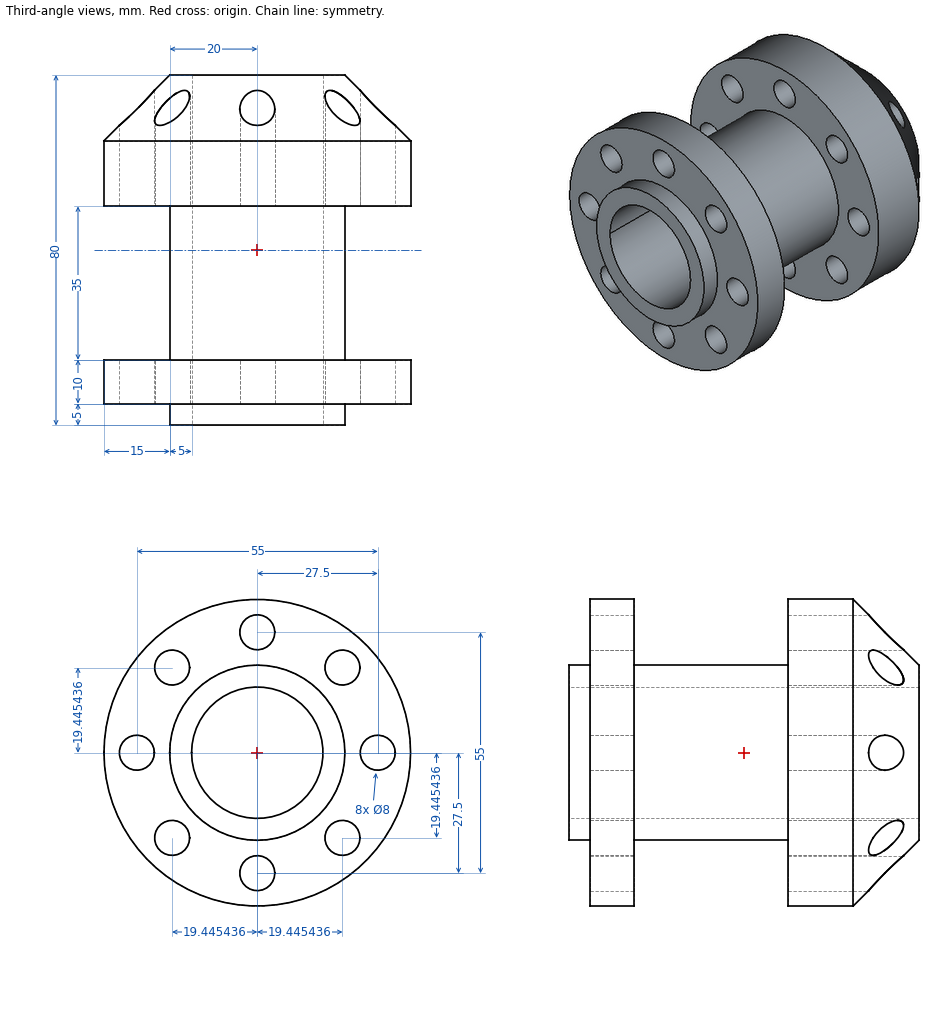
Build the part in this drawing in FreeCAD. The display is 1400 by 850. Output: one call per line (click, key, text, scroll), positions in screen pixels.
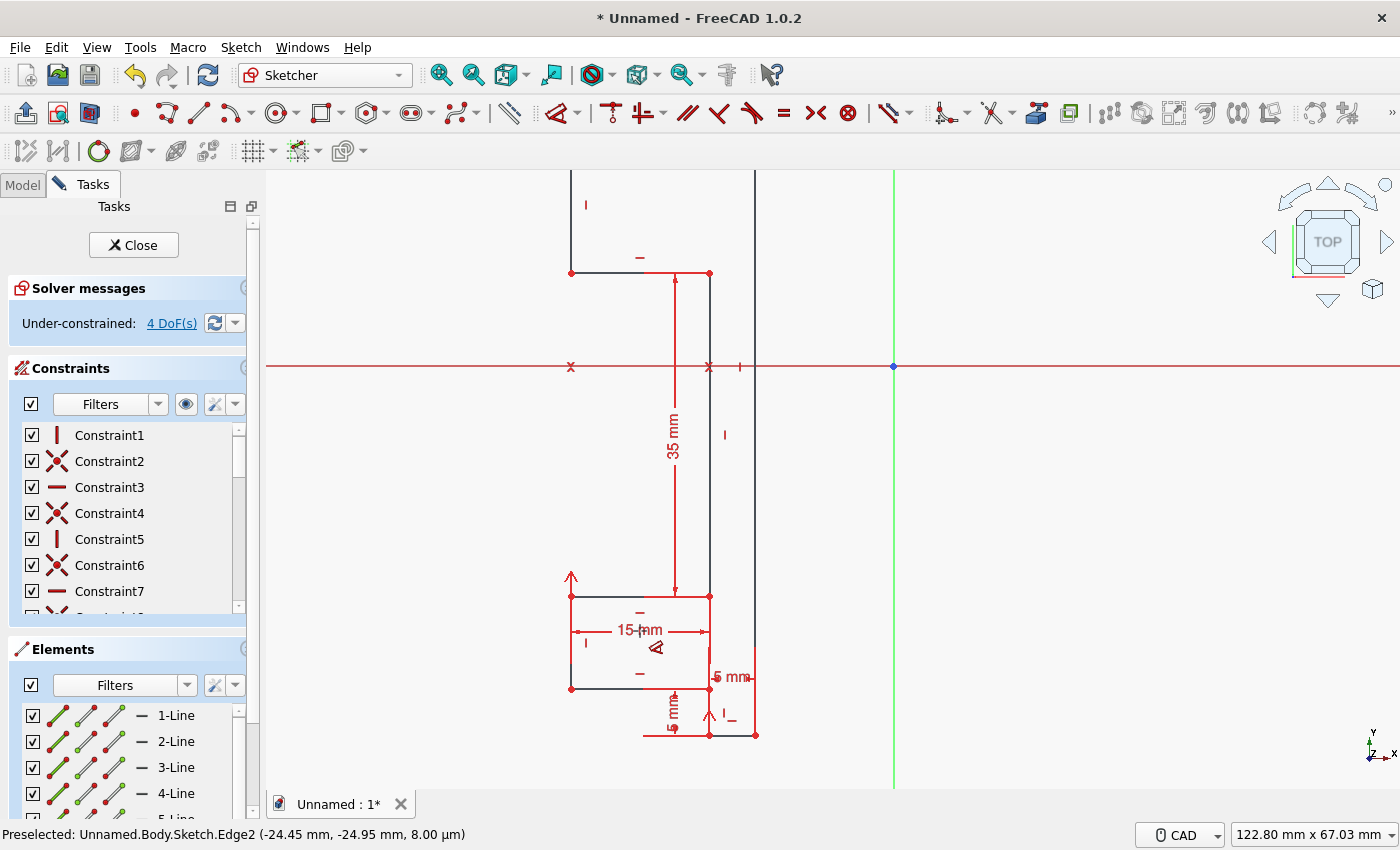
click(571, 624)
click(537, 643)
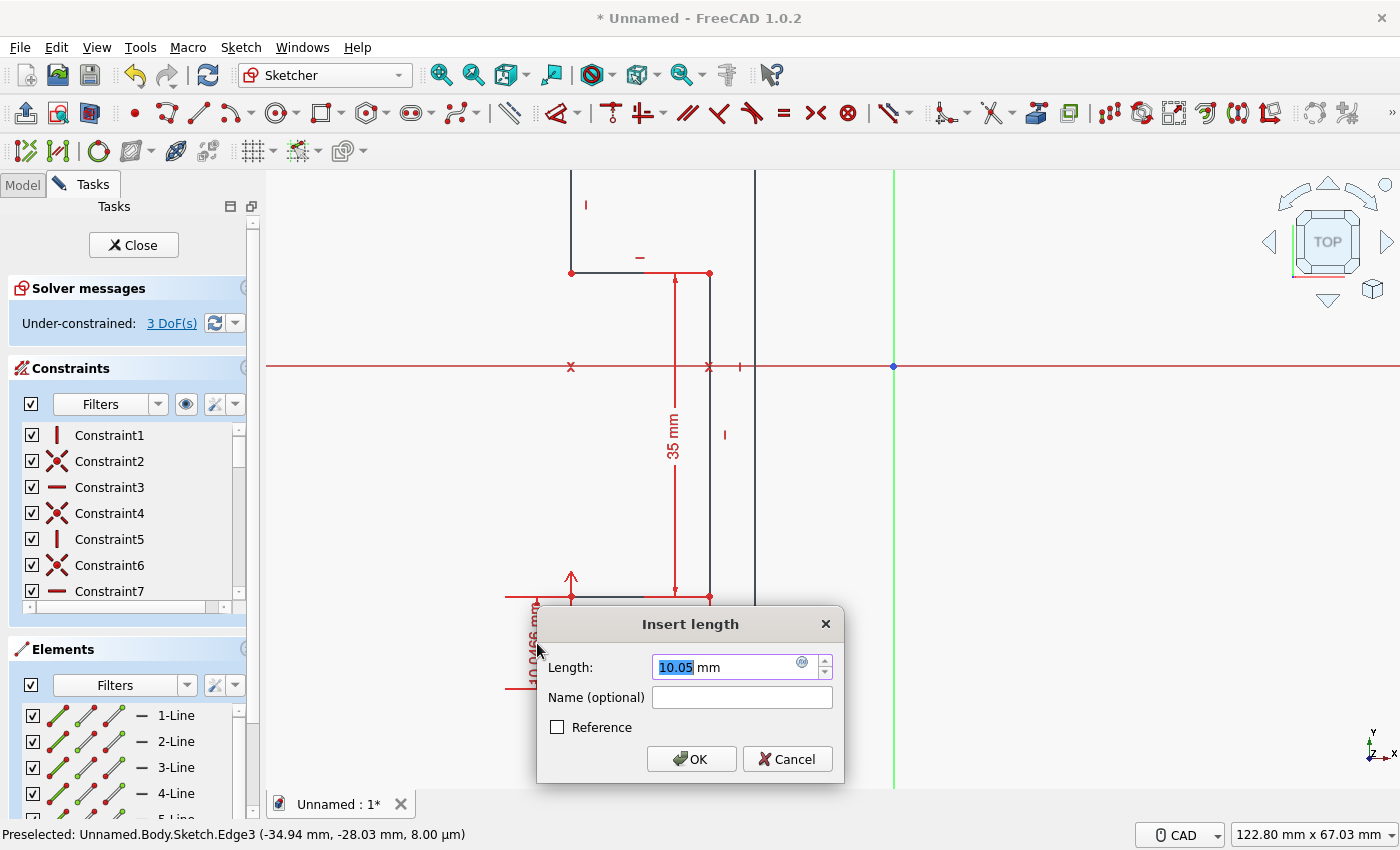
text(10)
key(Return)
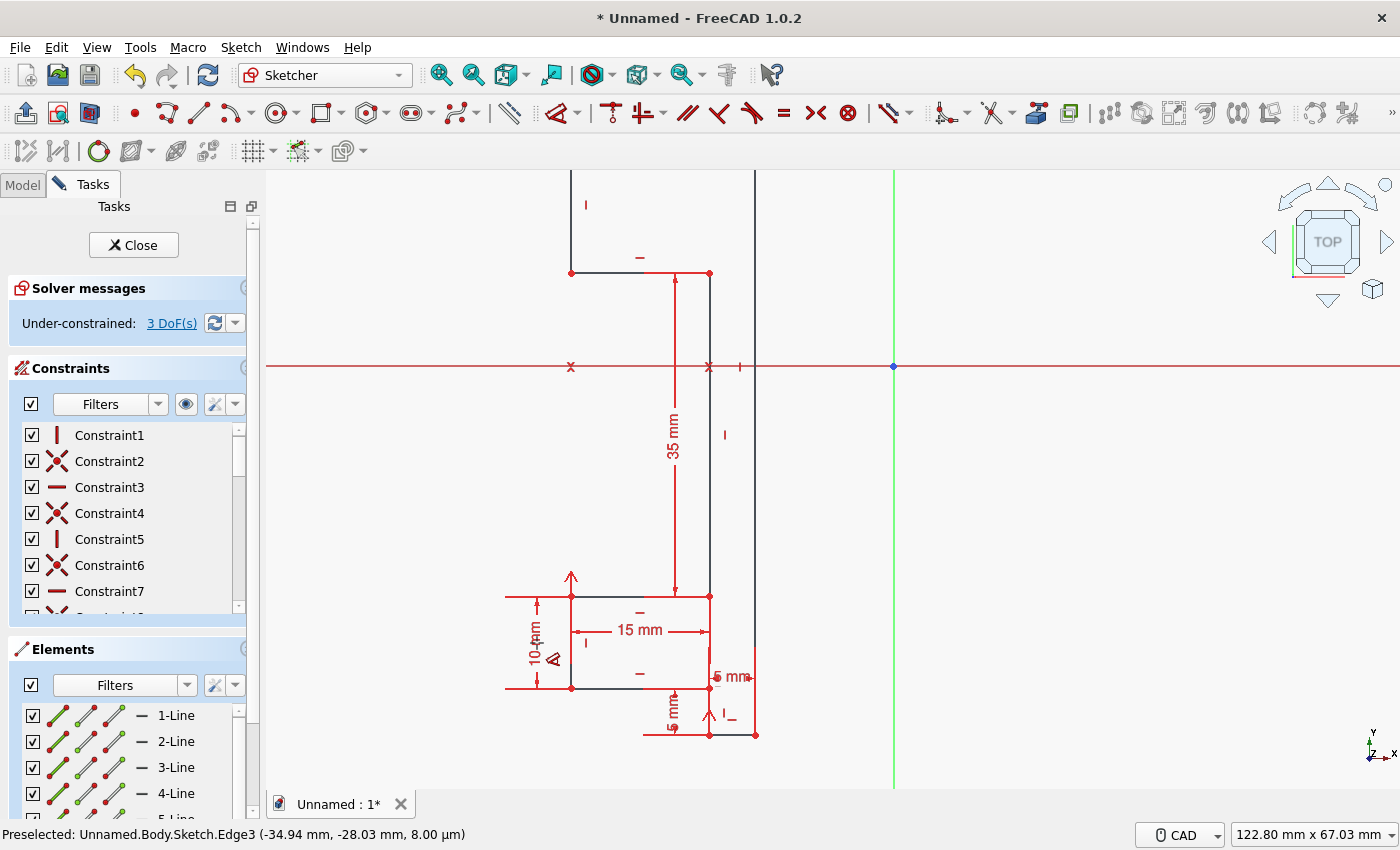
click(613, 689)
click(592, 723)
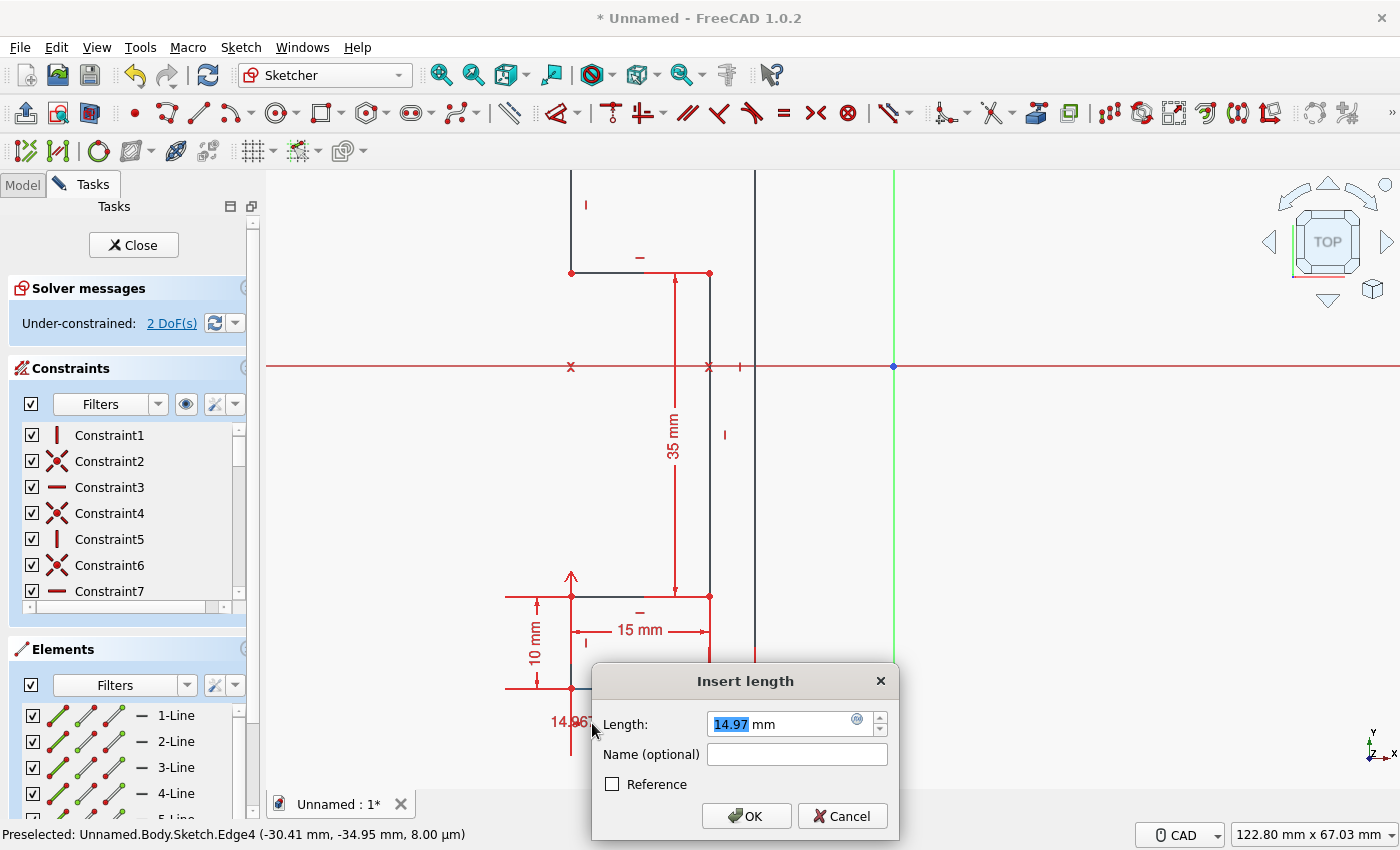
text(15)
key(Return)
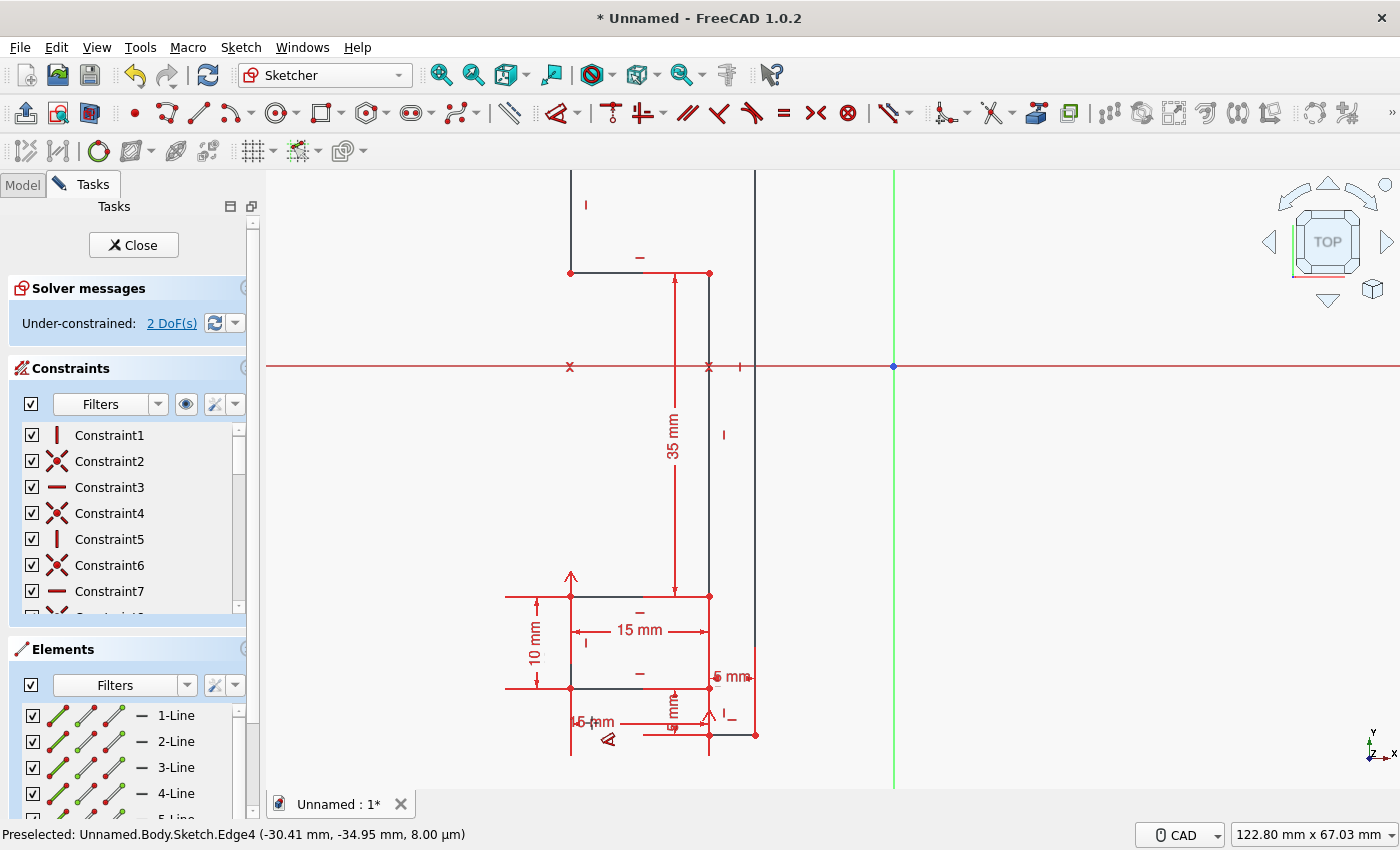
click(756, 514)
click(790, 467)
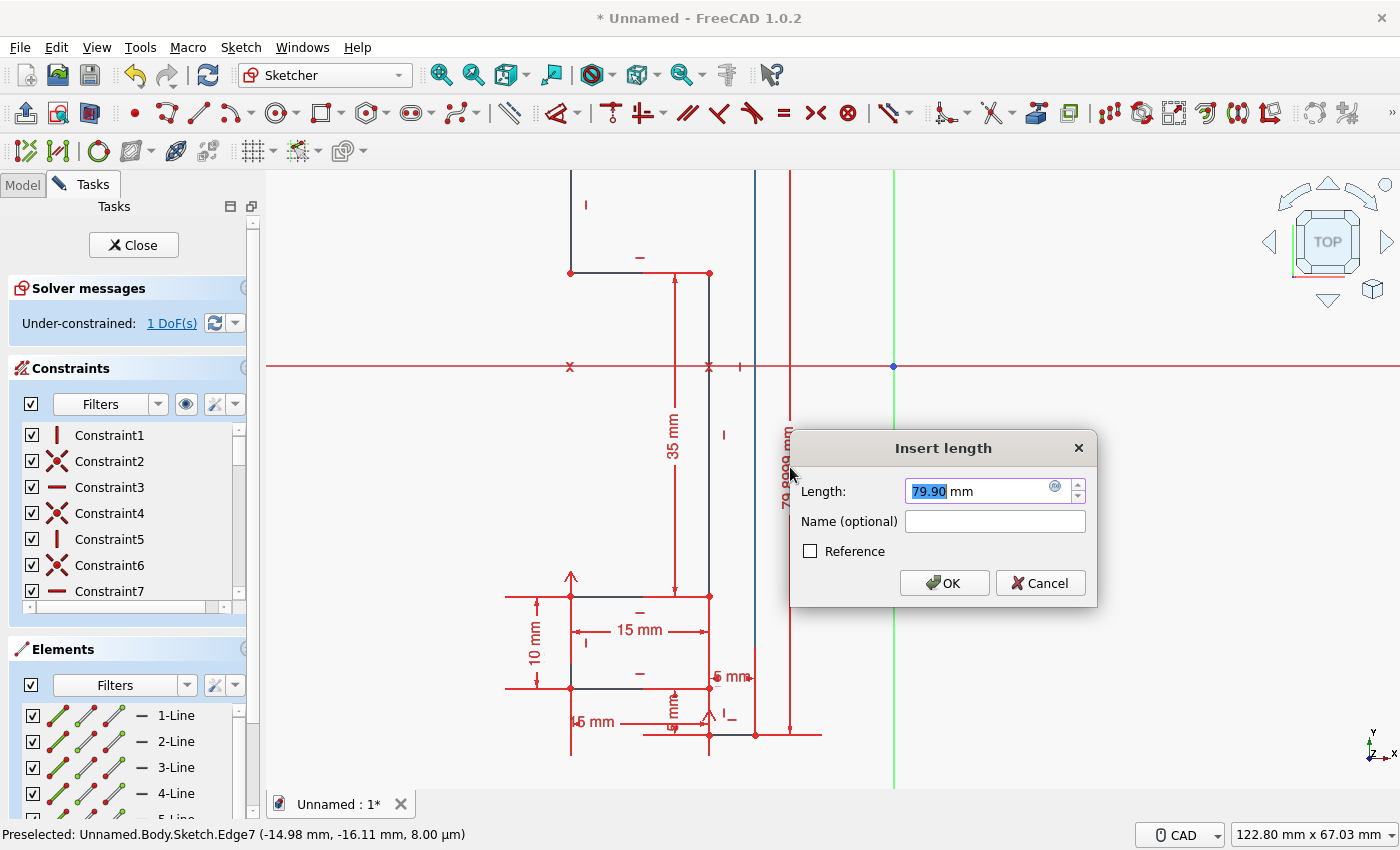
text(80)
key(Return)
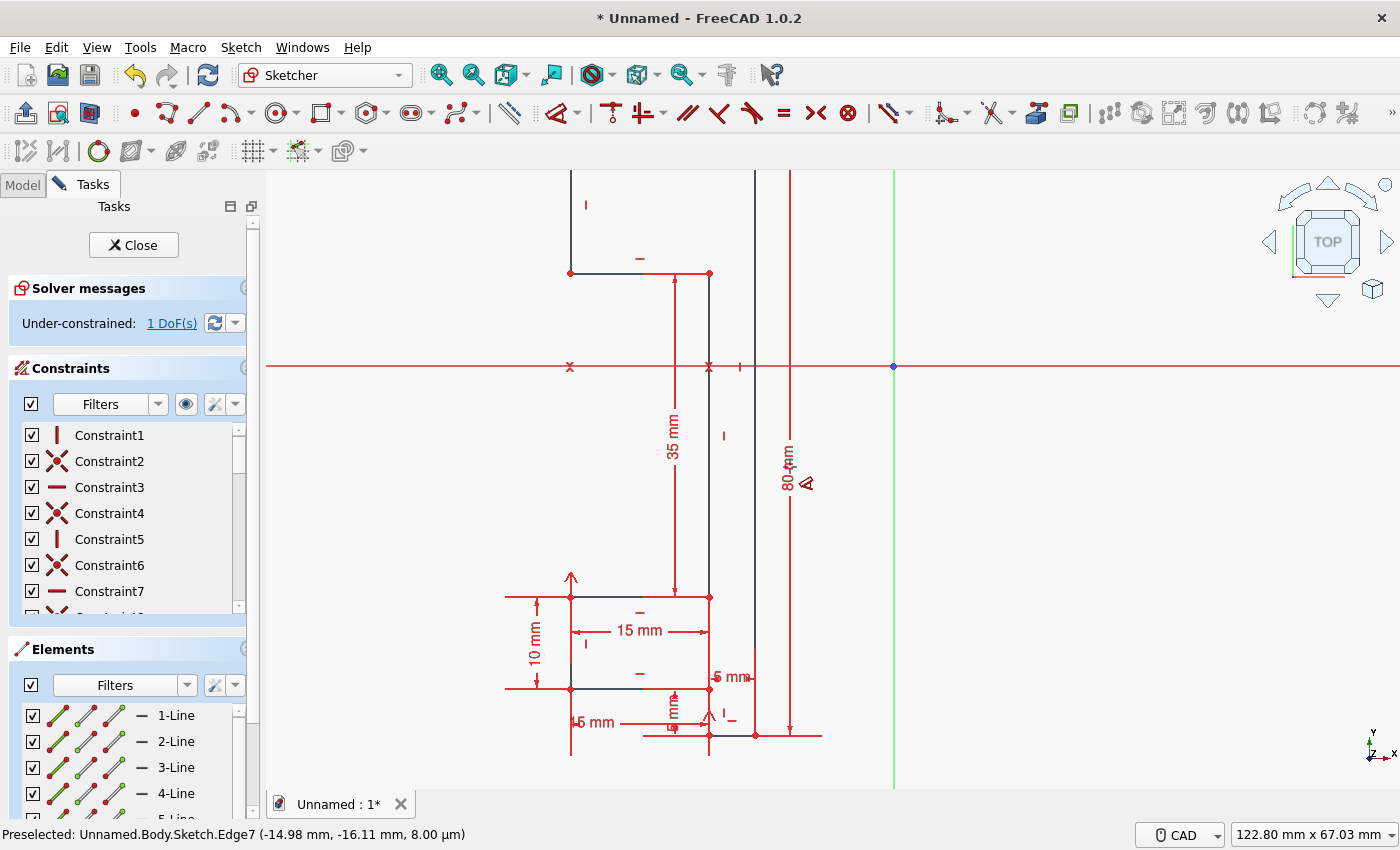
click(709, 274)
click(802, 240)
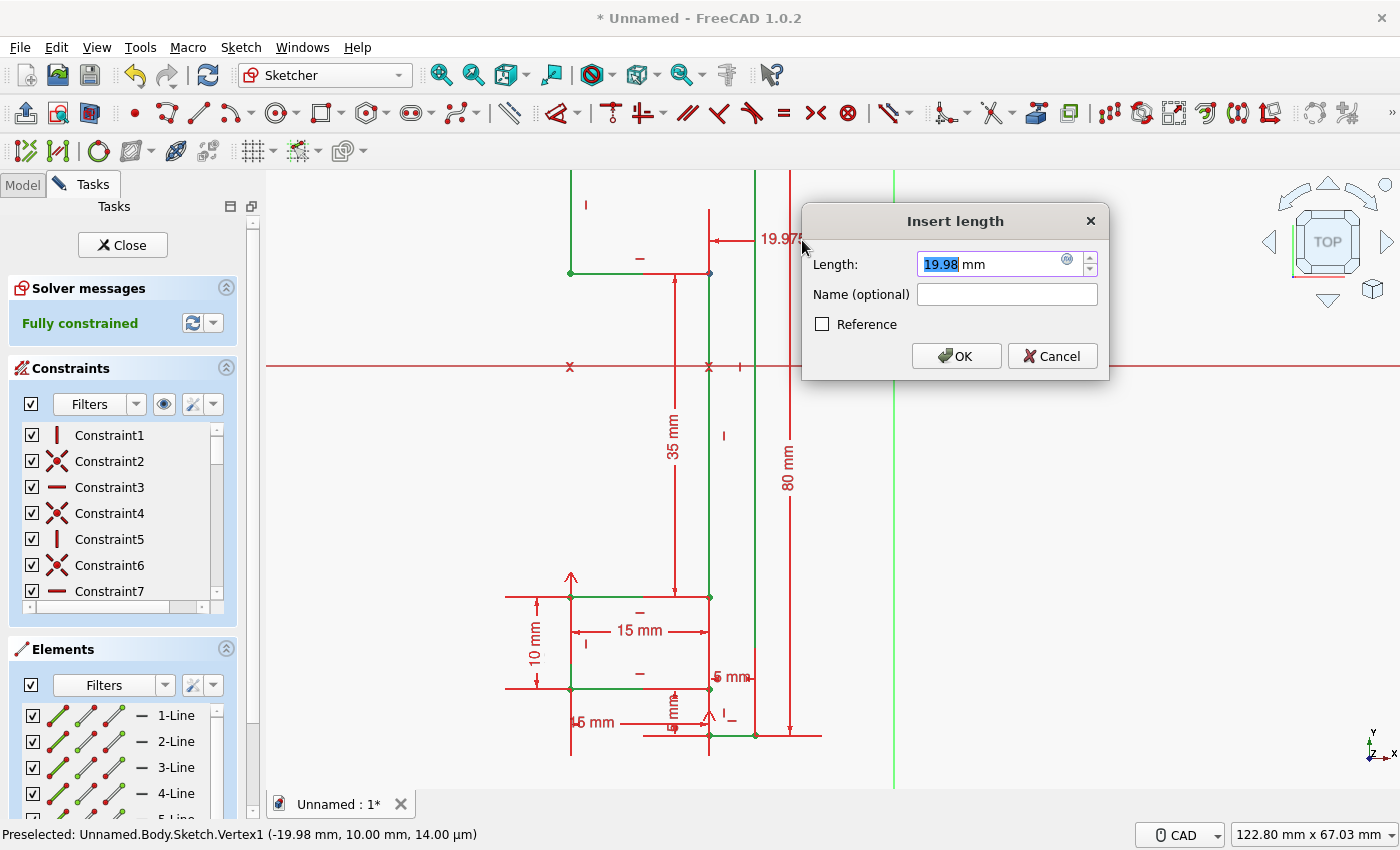
text(20)
key(Return)
key(Escape)